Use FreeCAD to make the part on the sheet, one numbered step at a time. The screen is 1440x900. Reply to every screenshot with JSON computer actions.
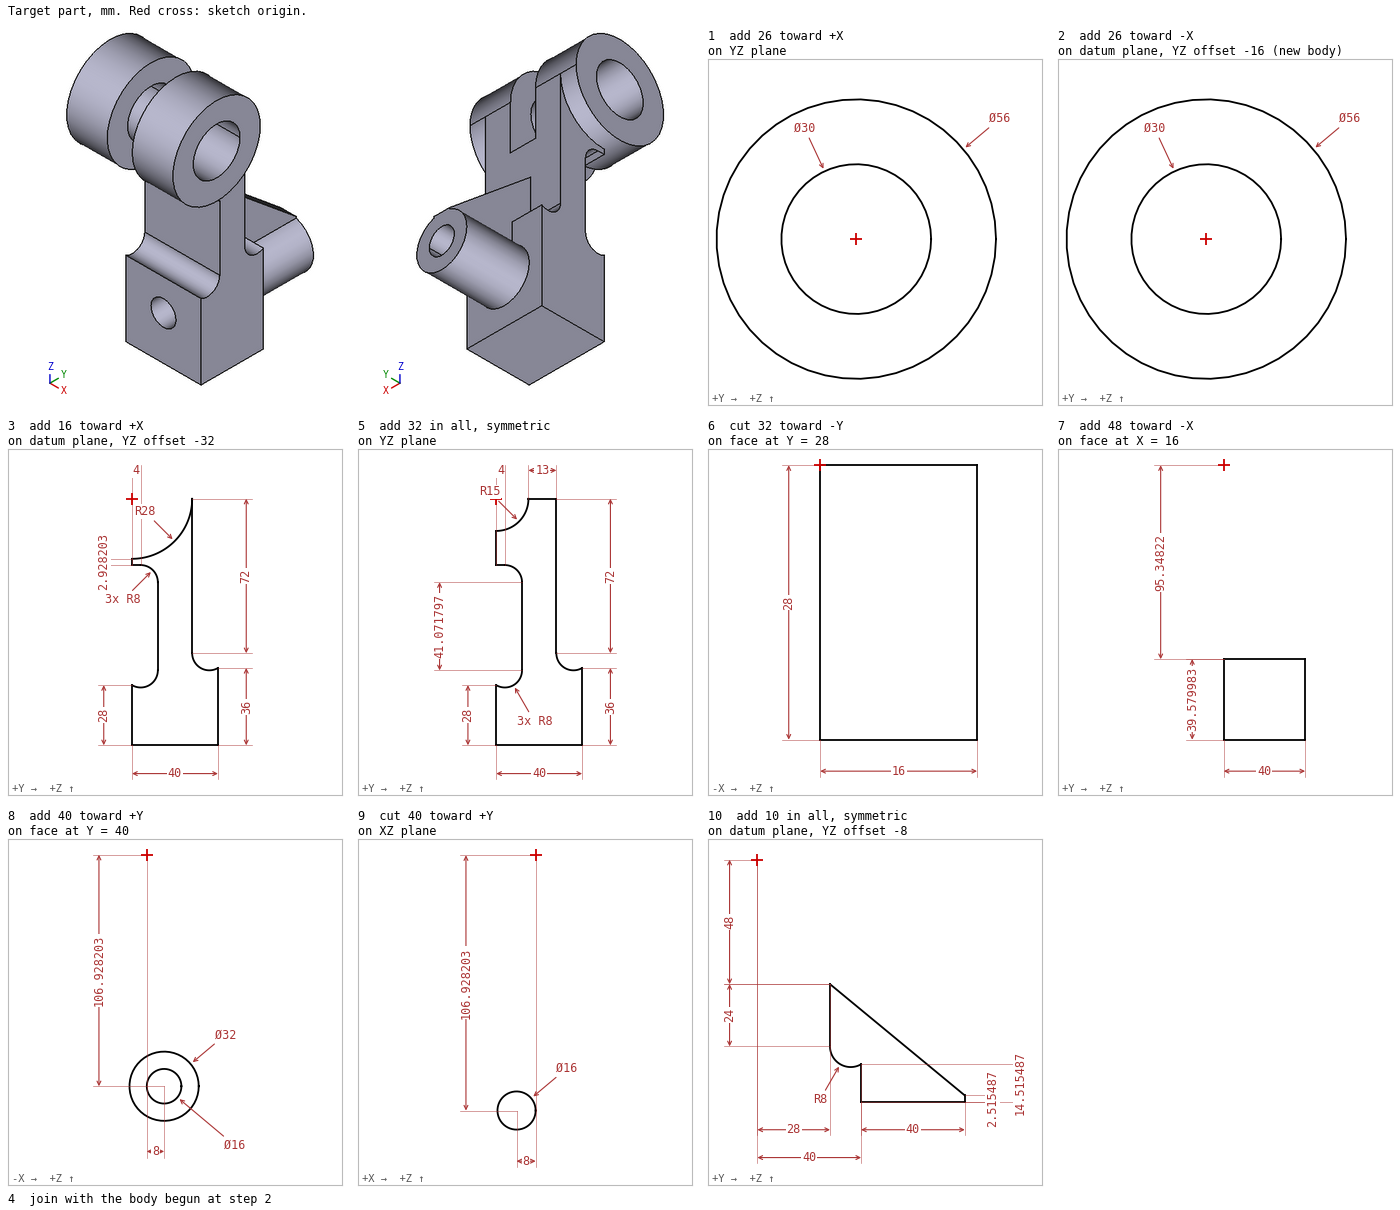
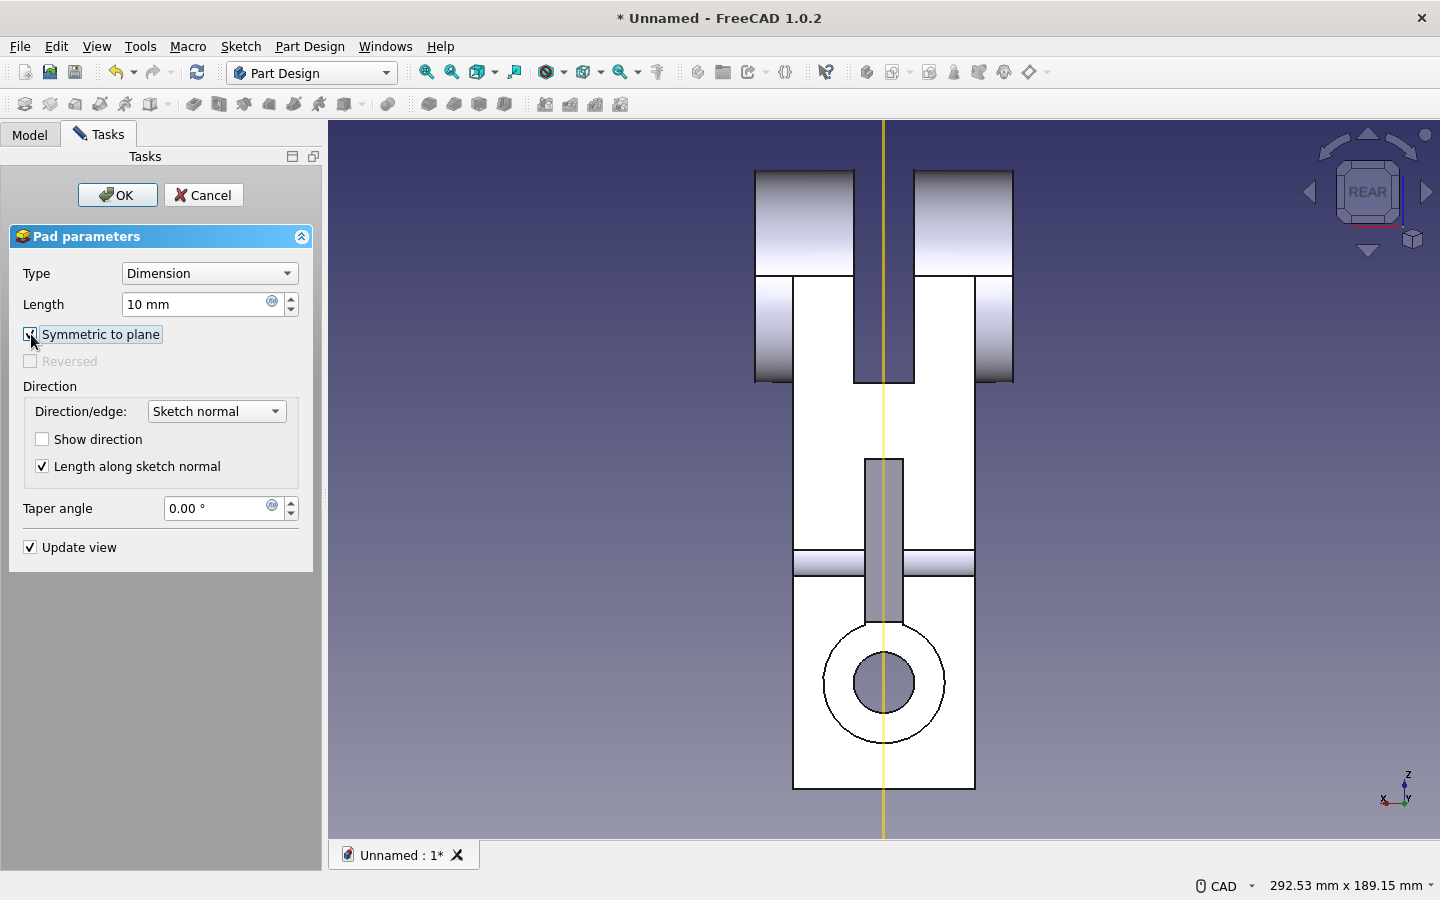
{"action": "left_click", "coordinate": [118, 195]}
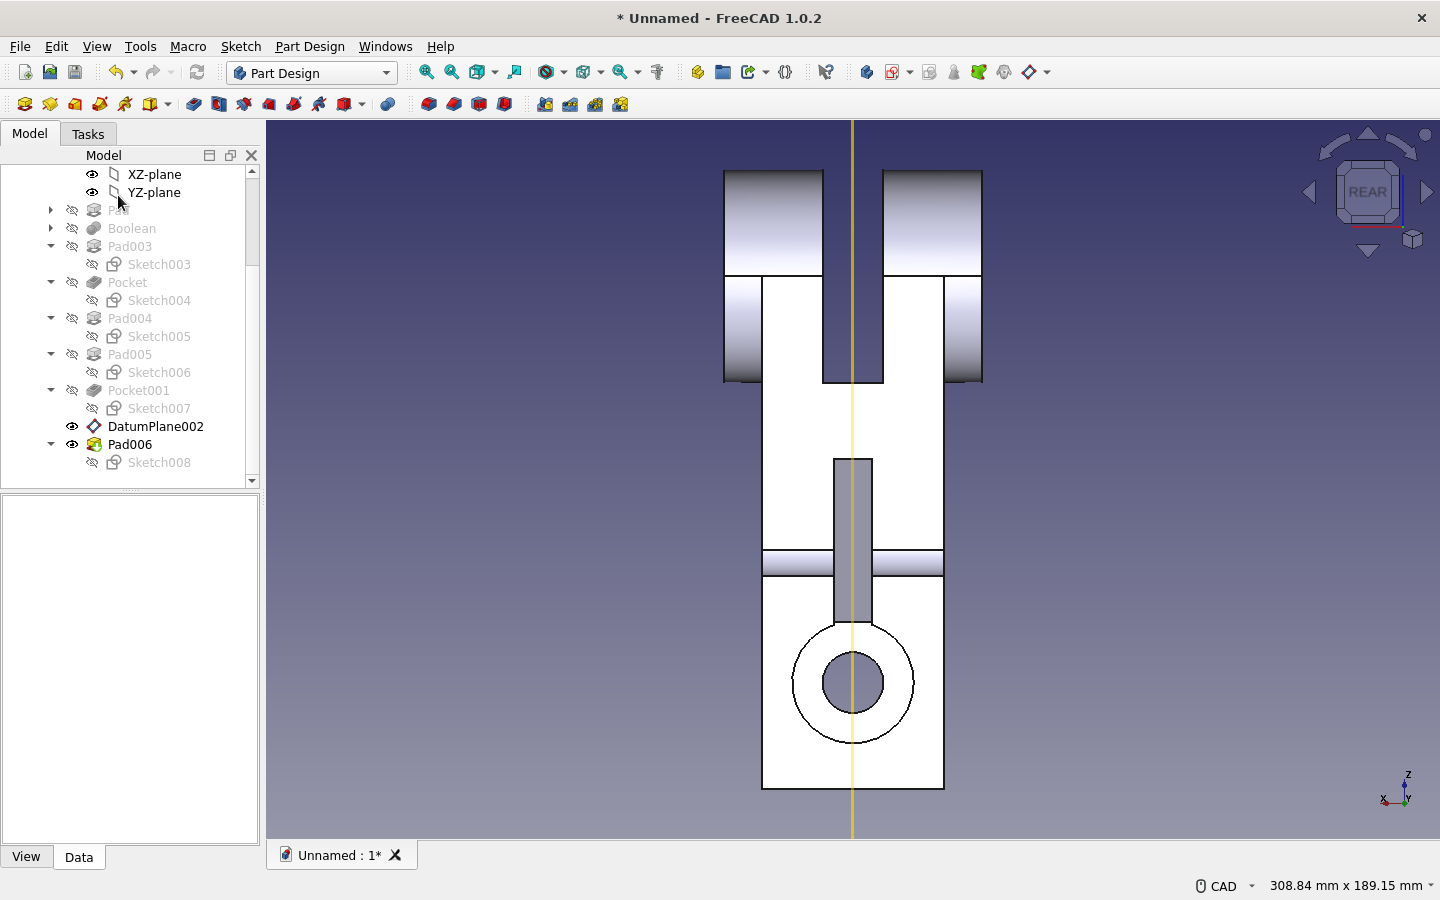
{"action": "left_click", "coordinate": [117, 426]}
{"action": "key", "text": "space"}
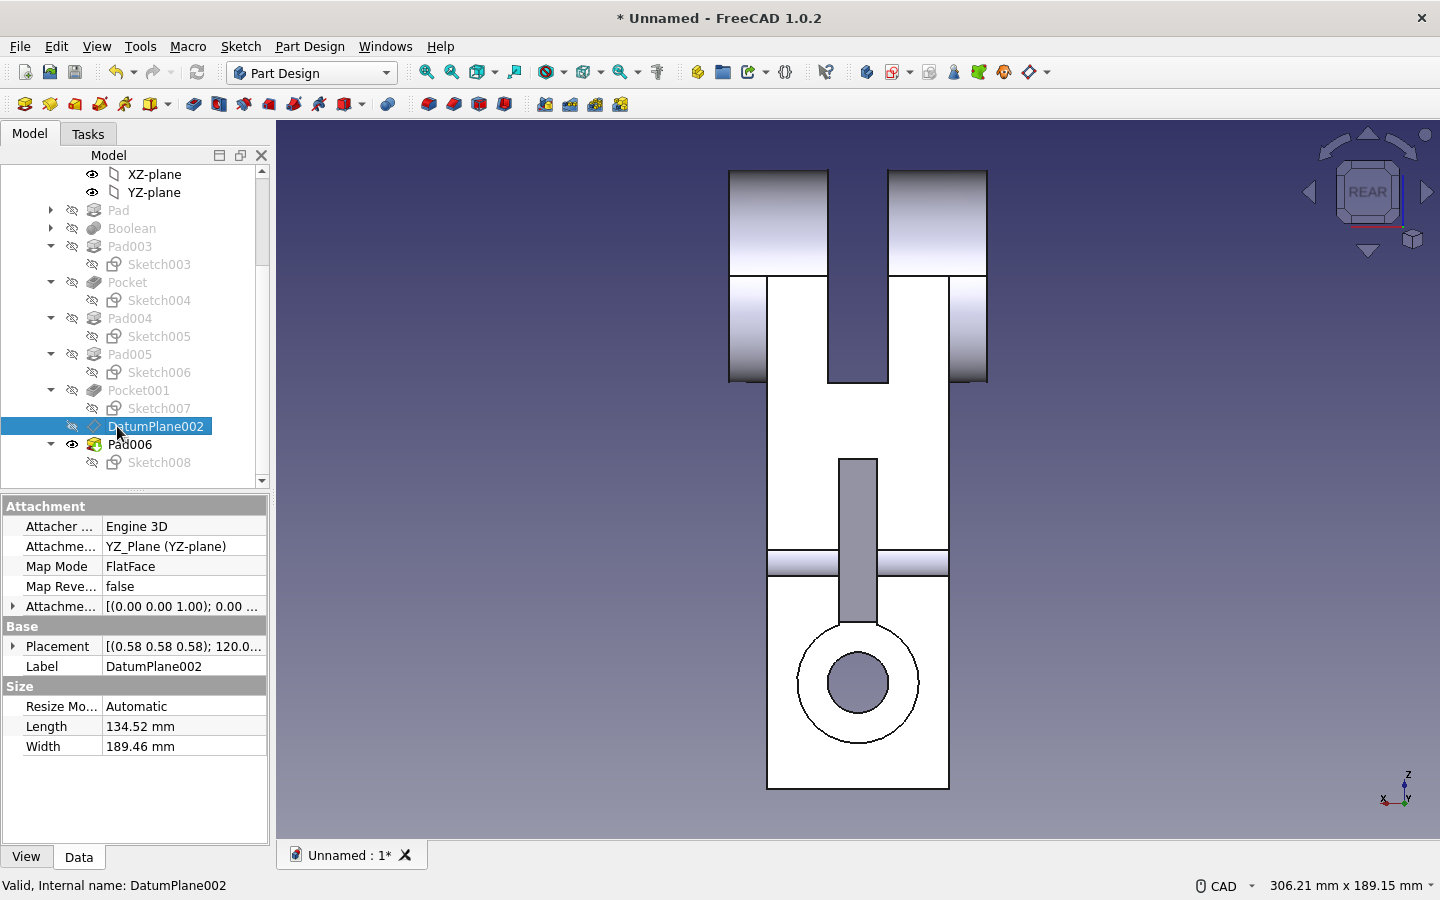
{"action": "key", "text": "0"}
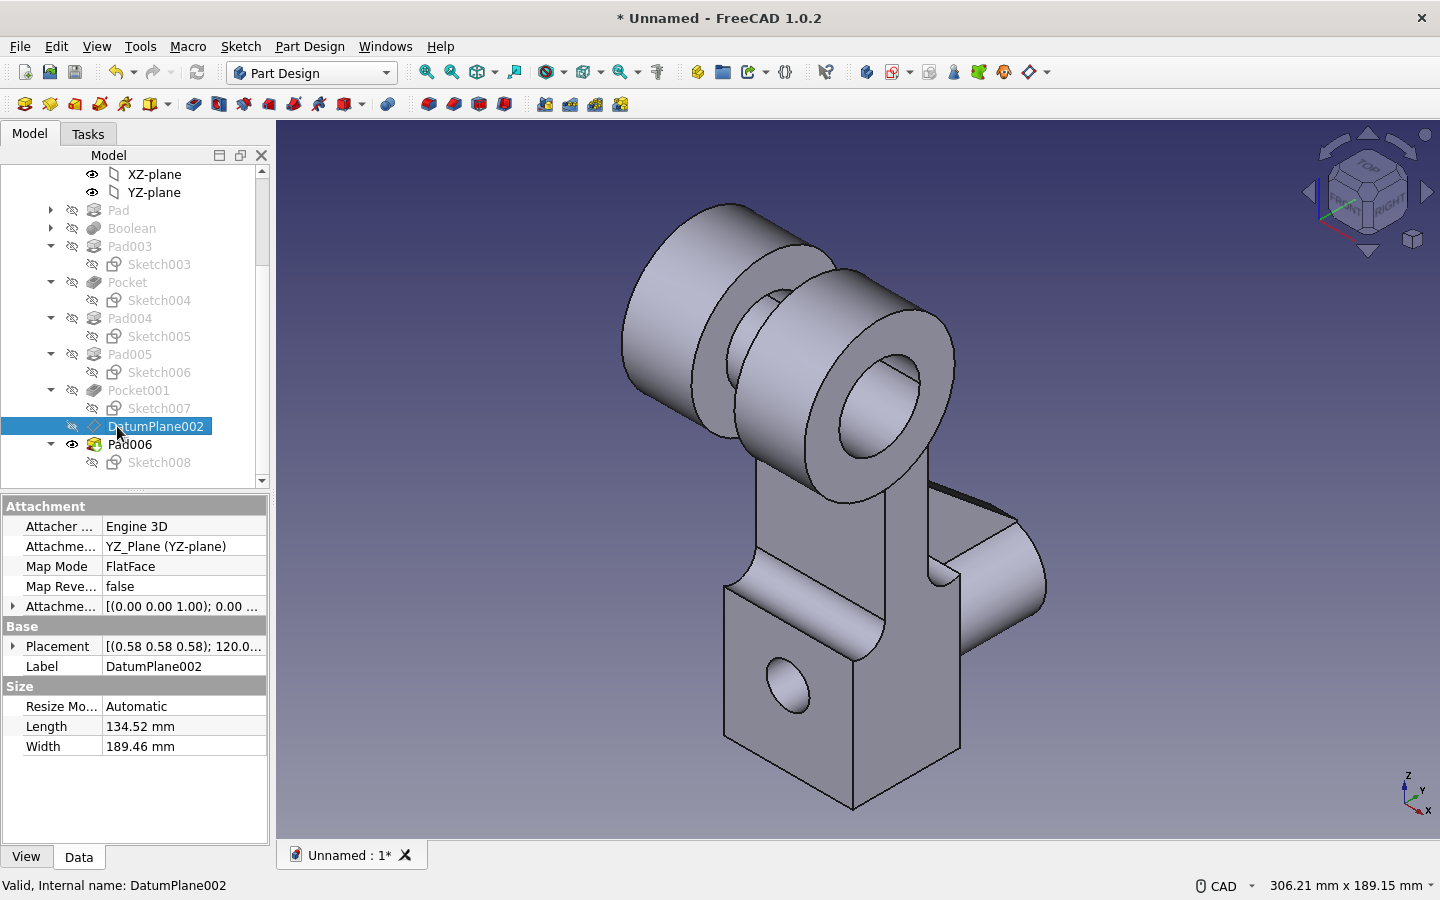
{"action": "key", "text": "v f"}